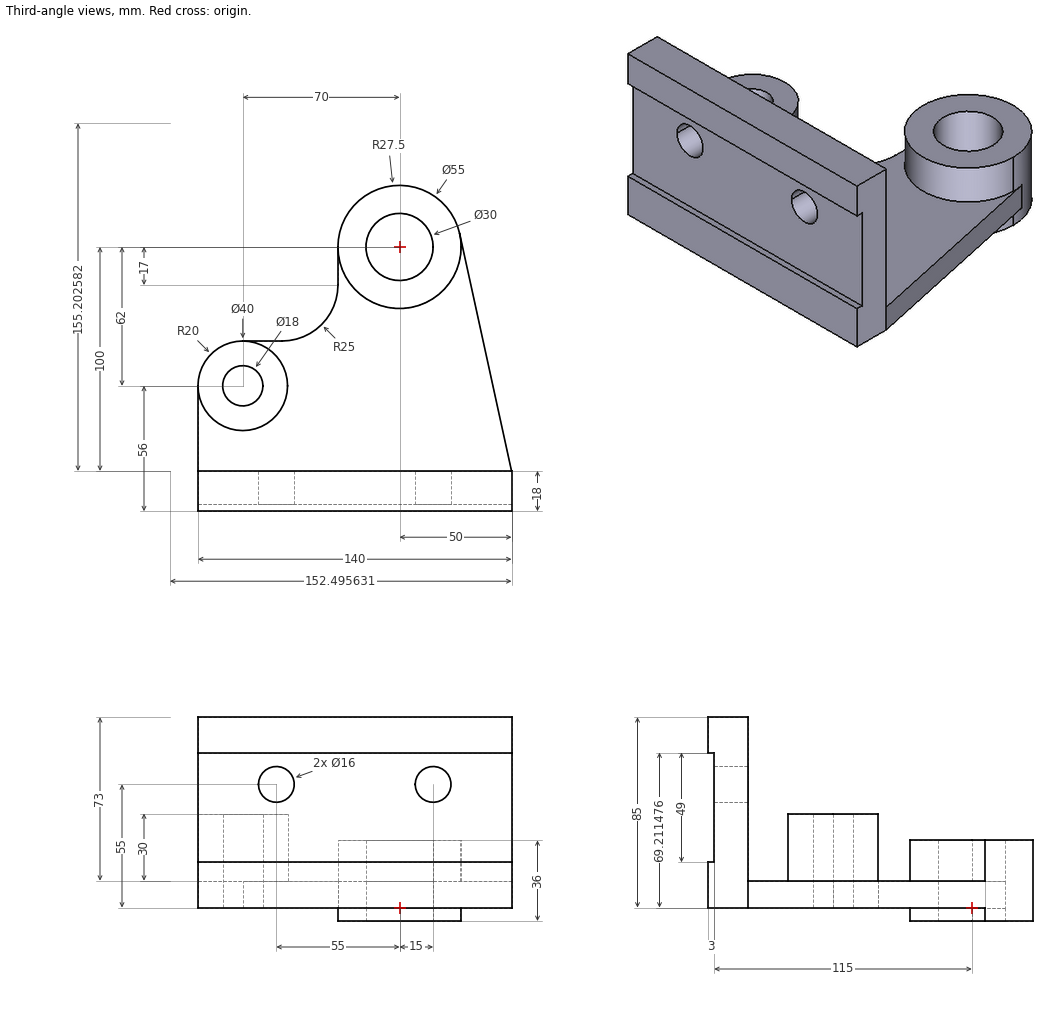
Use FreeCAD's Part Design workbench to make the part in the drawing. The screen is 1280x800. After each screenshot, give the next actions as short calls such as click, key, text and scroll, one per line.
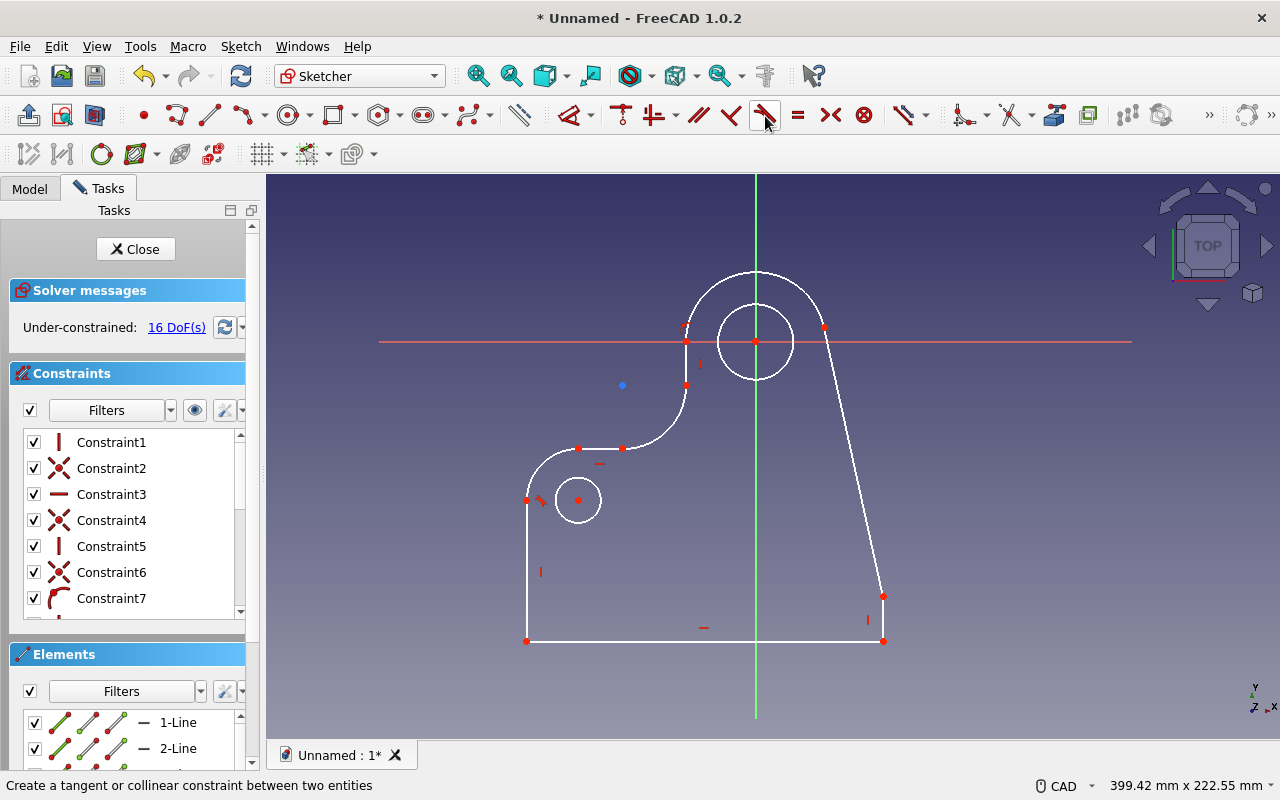
click(865, 516)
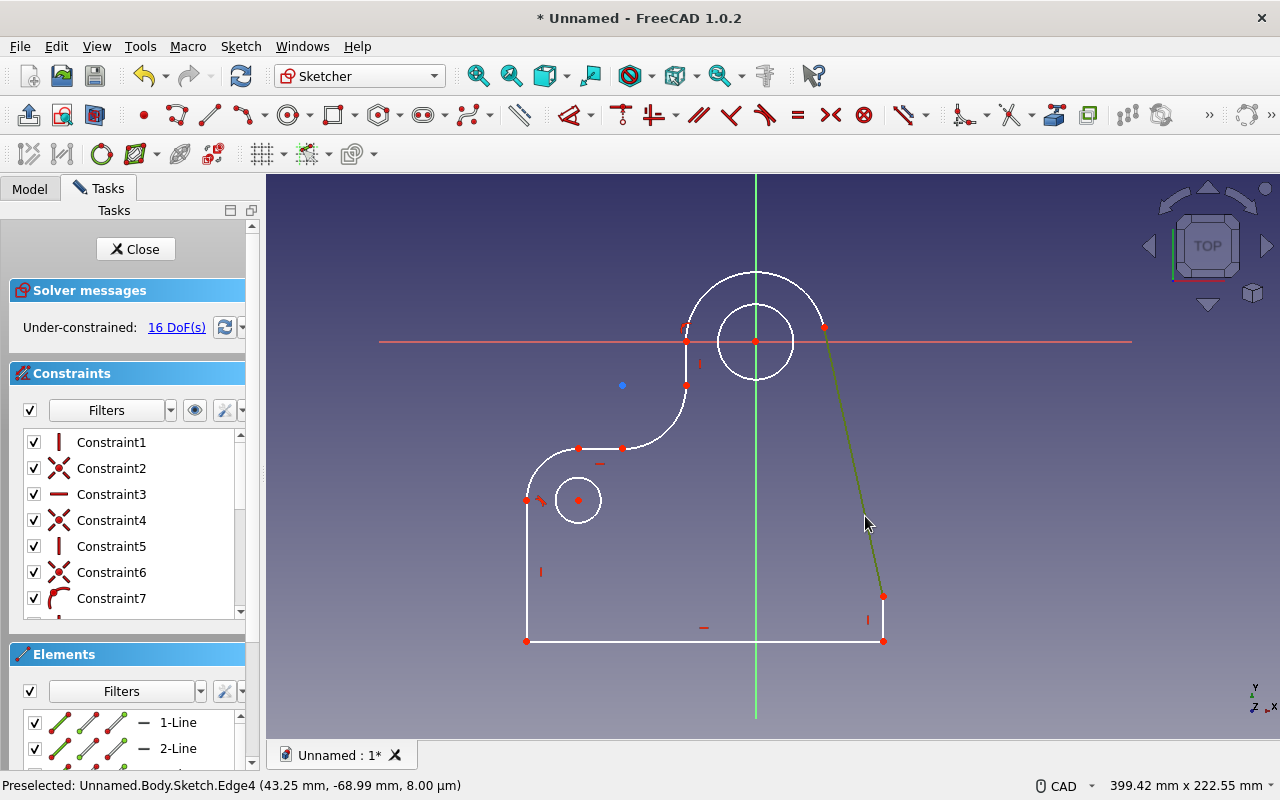
click(788, 280)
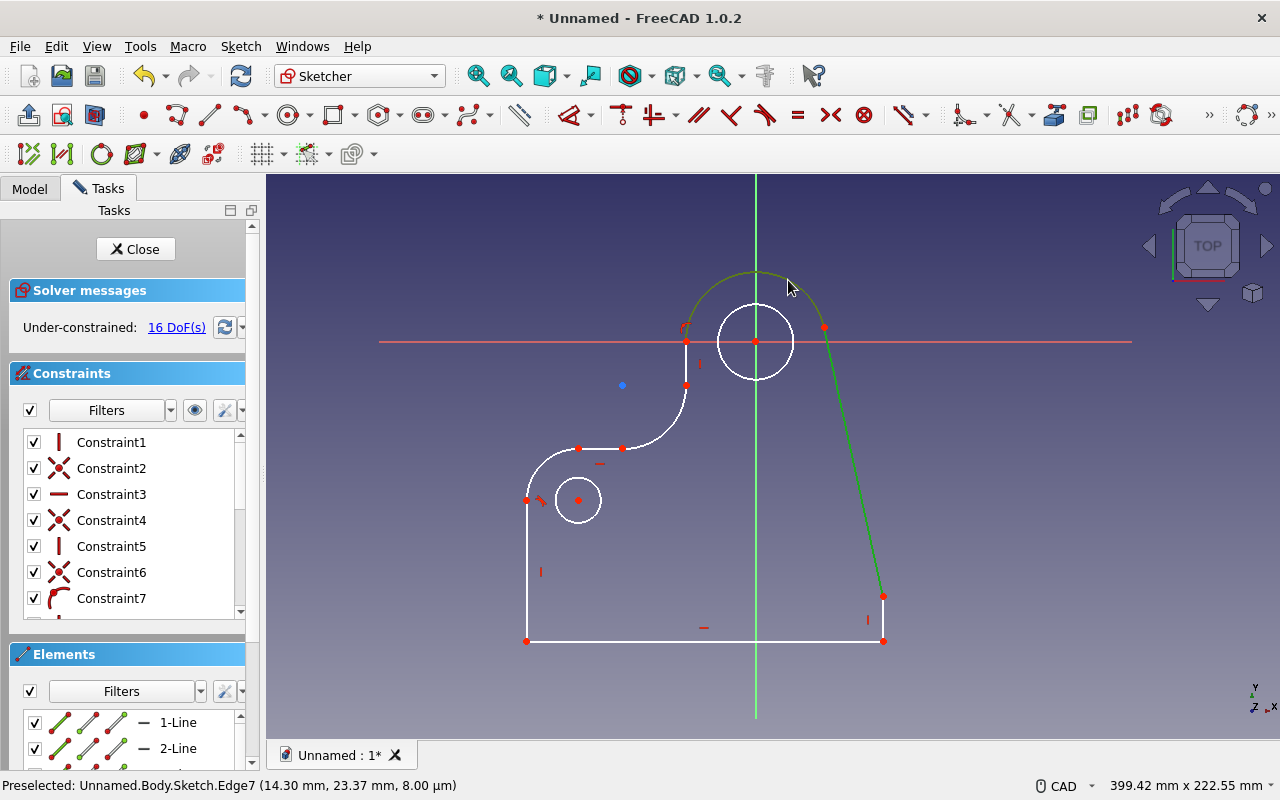
click(765, 116)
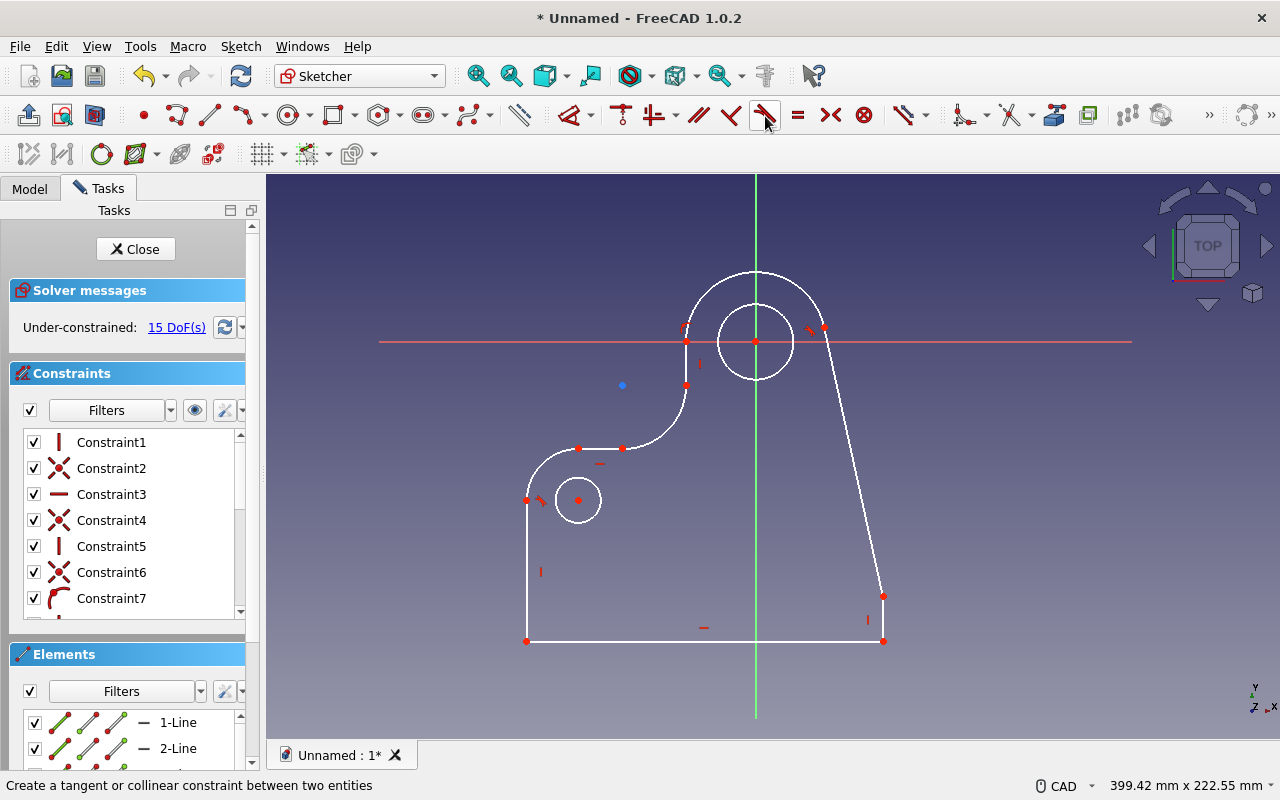
click(686, 355)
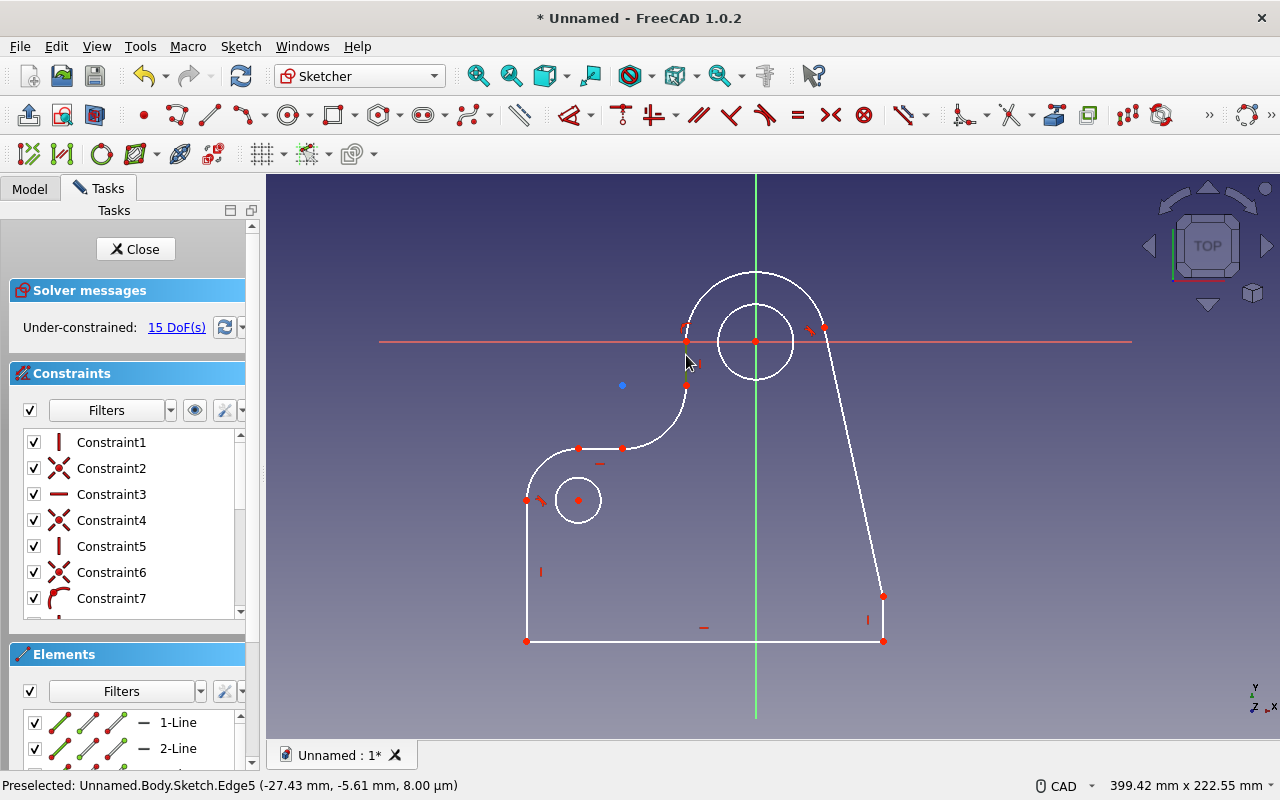
click(651, 442)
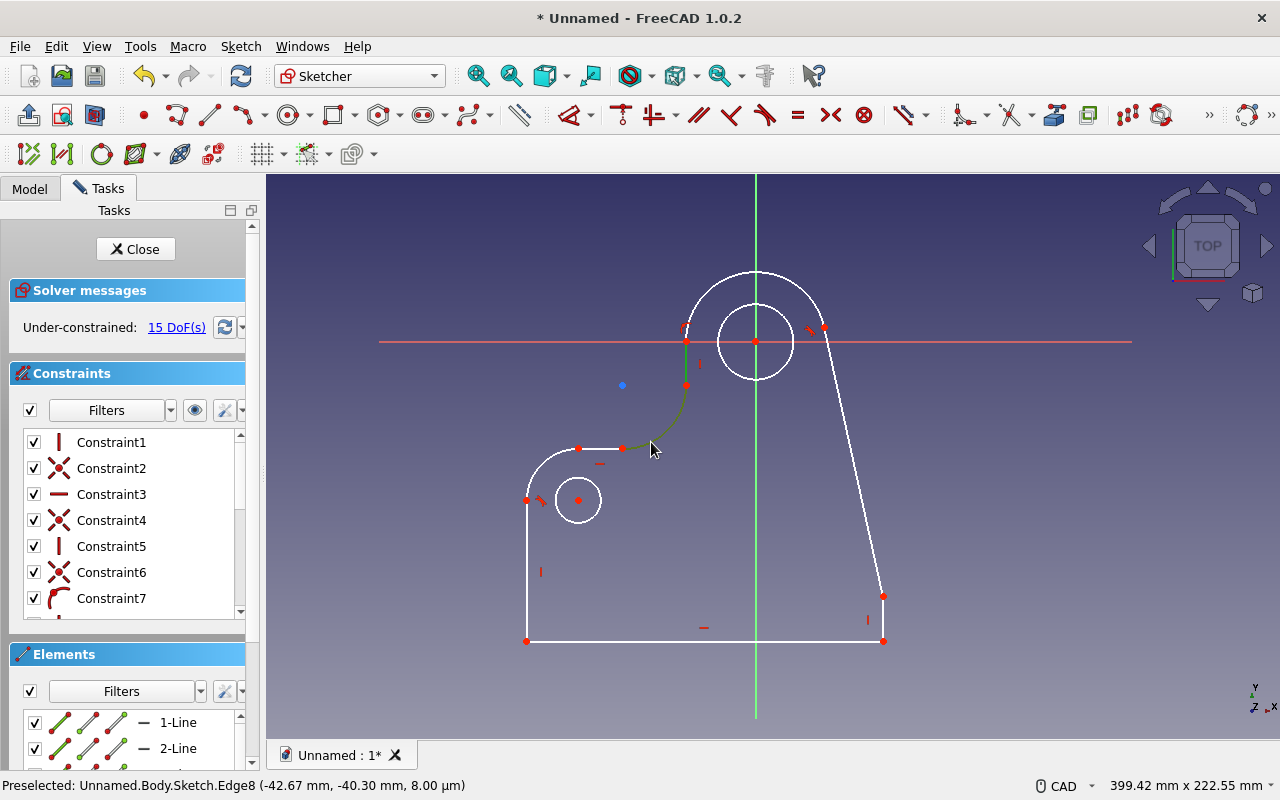
click(765, 116)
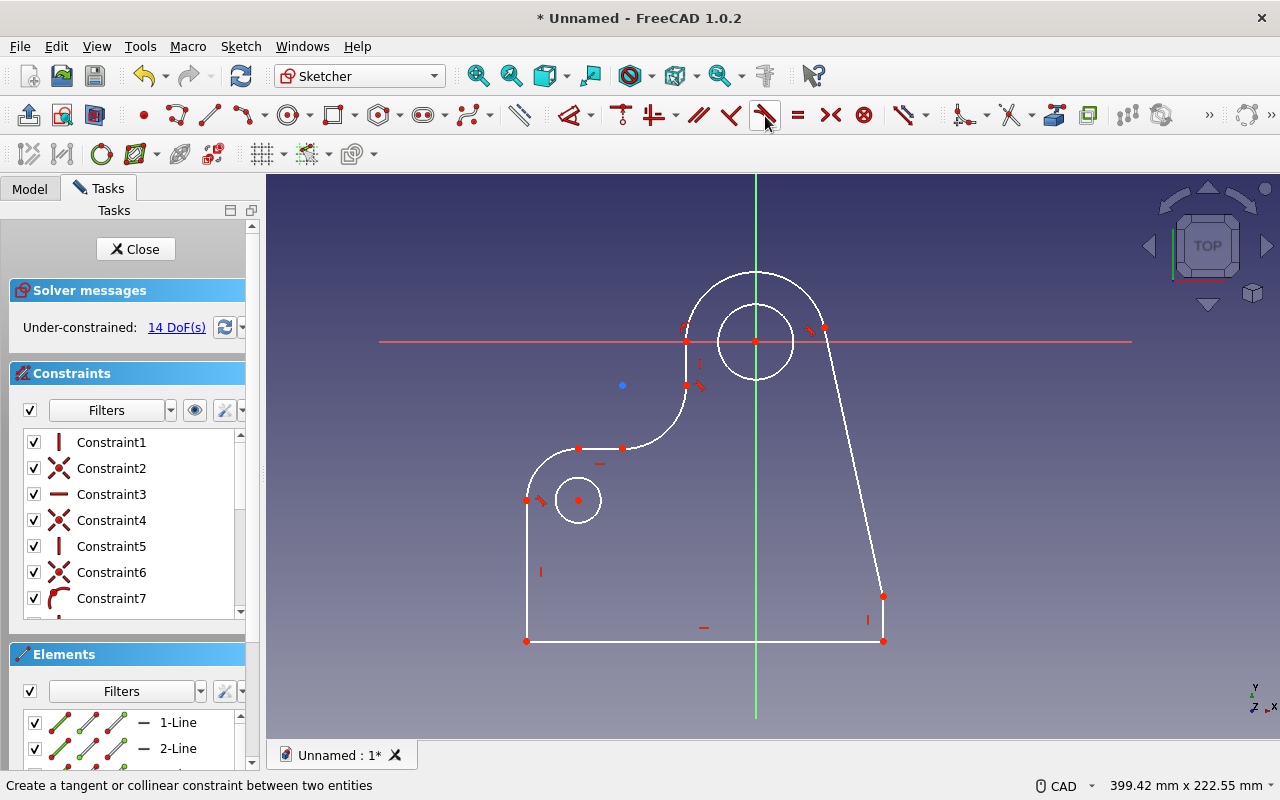
click(609, 449)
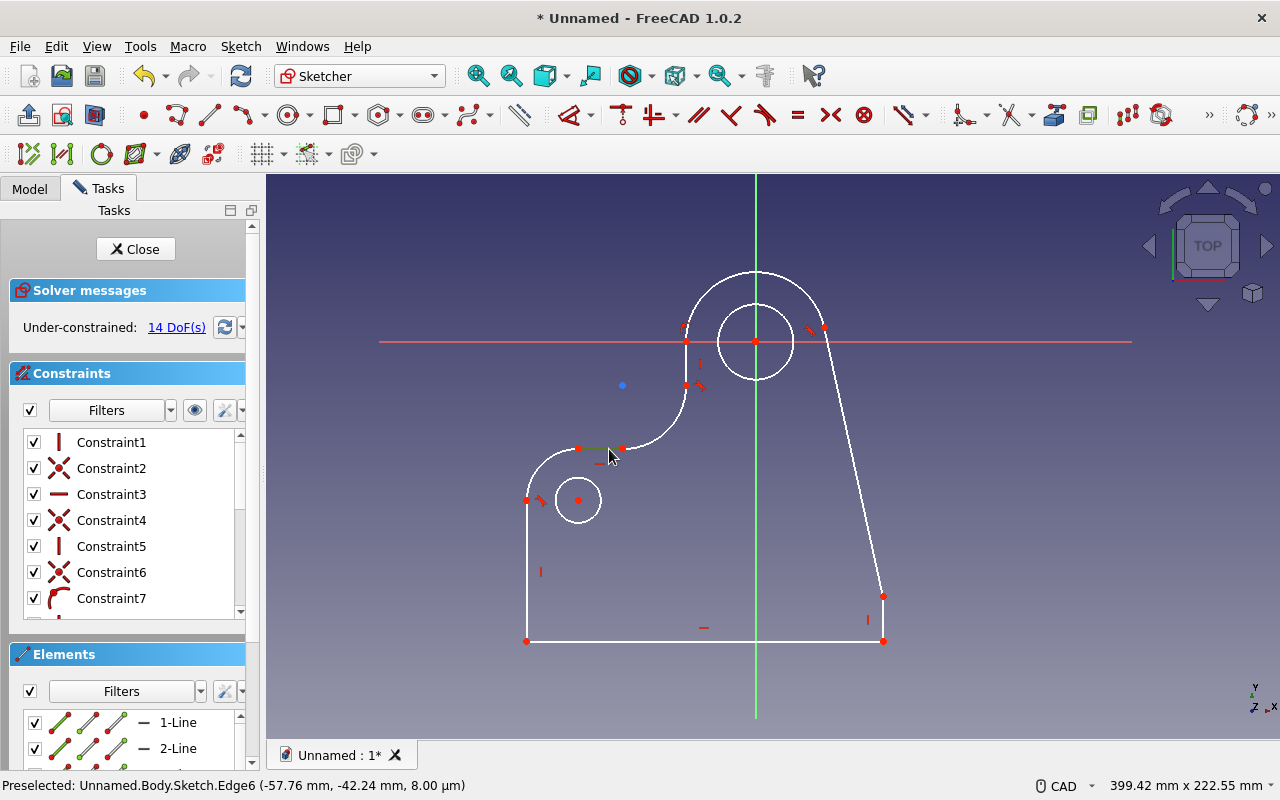
click(651, 442)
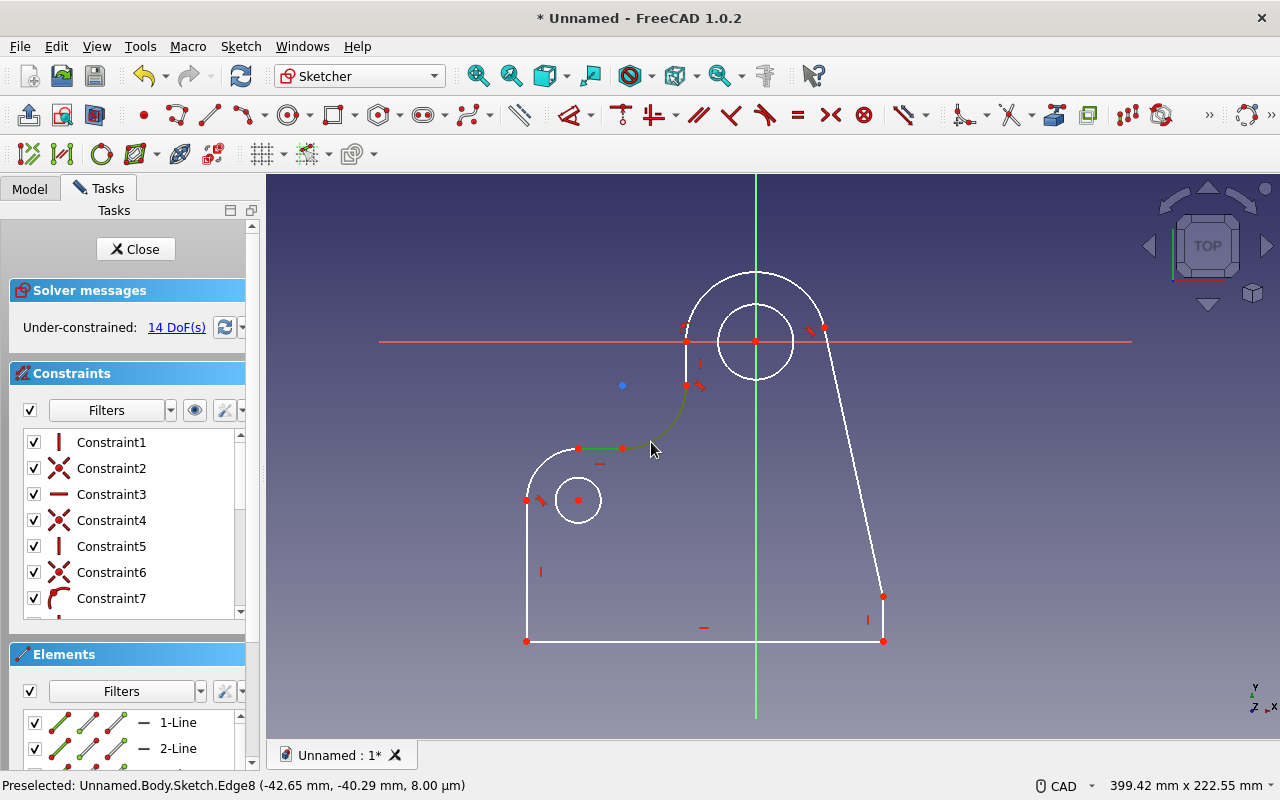
click(765, 116)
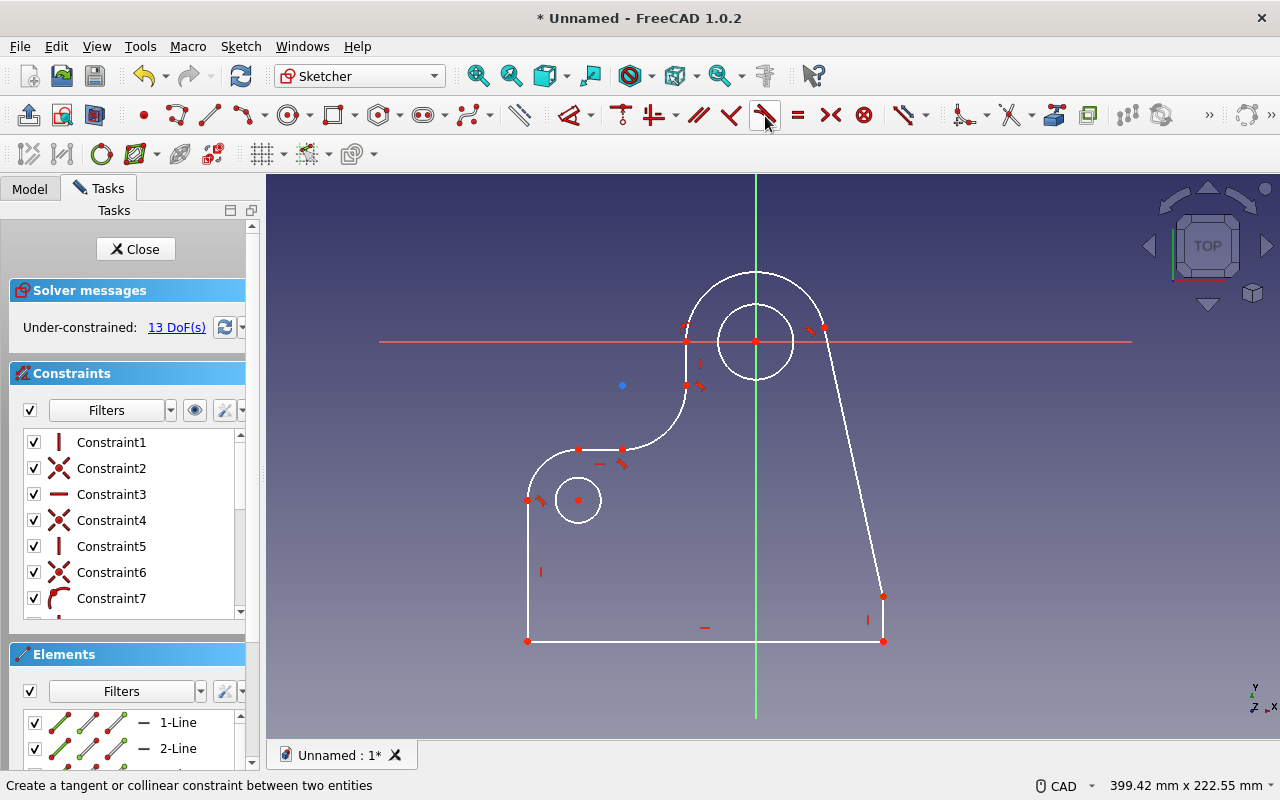
click(609, 450)